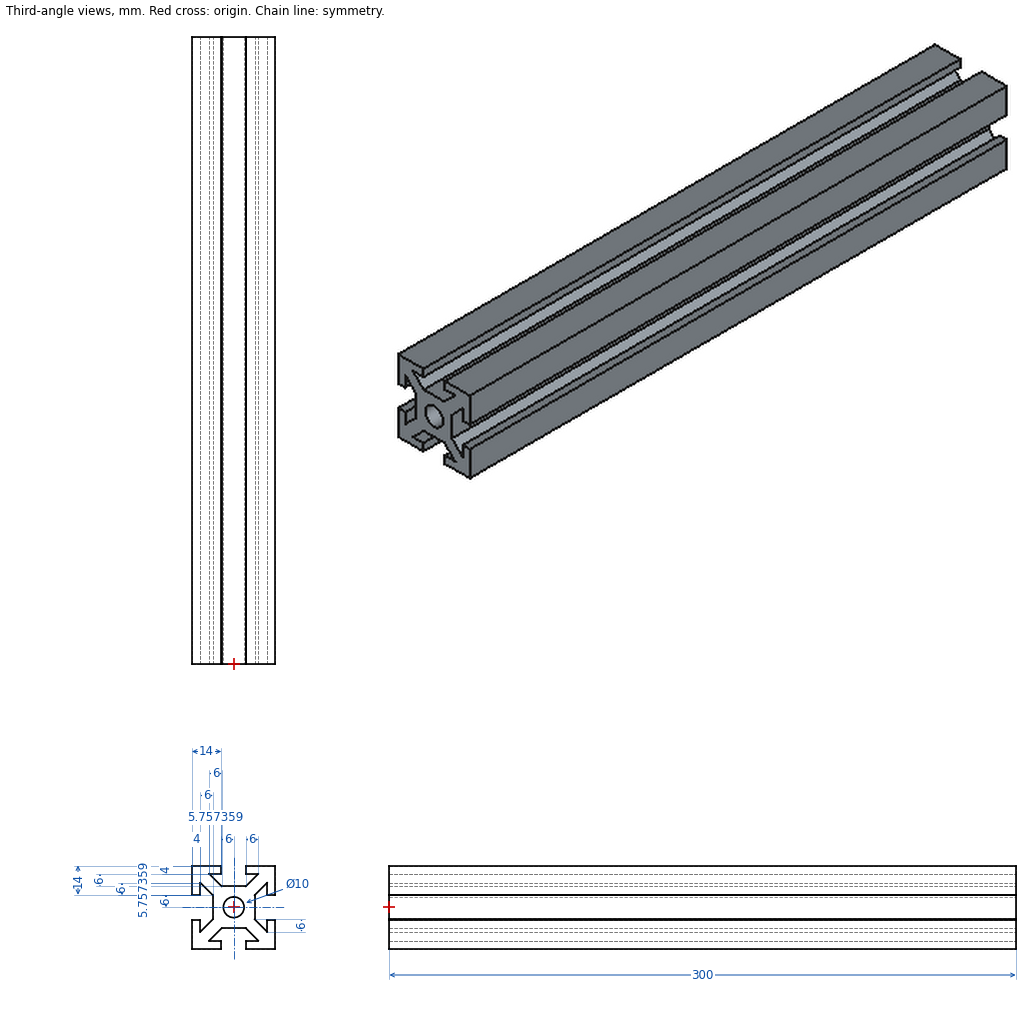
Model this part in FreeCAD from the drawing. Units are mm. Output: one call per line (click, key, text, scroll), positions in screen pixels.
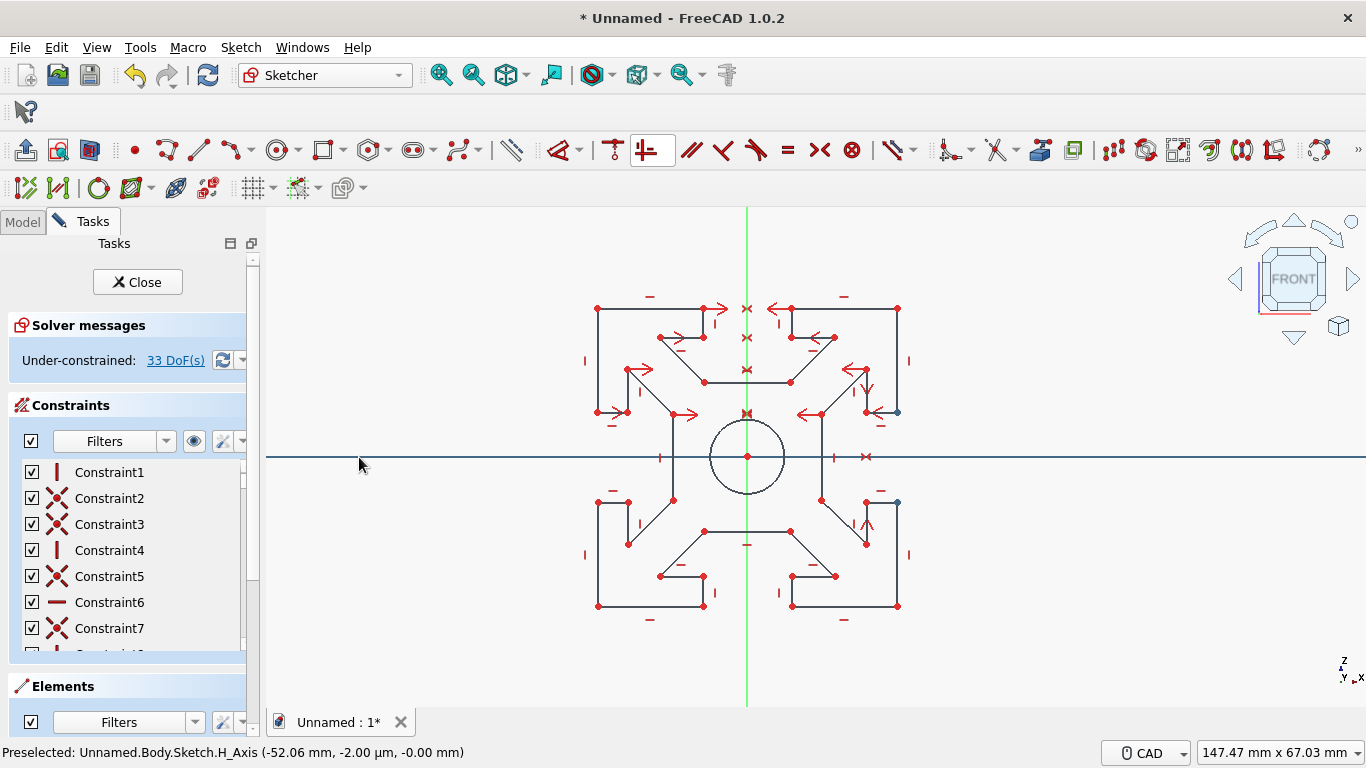
key(s)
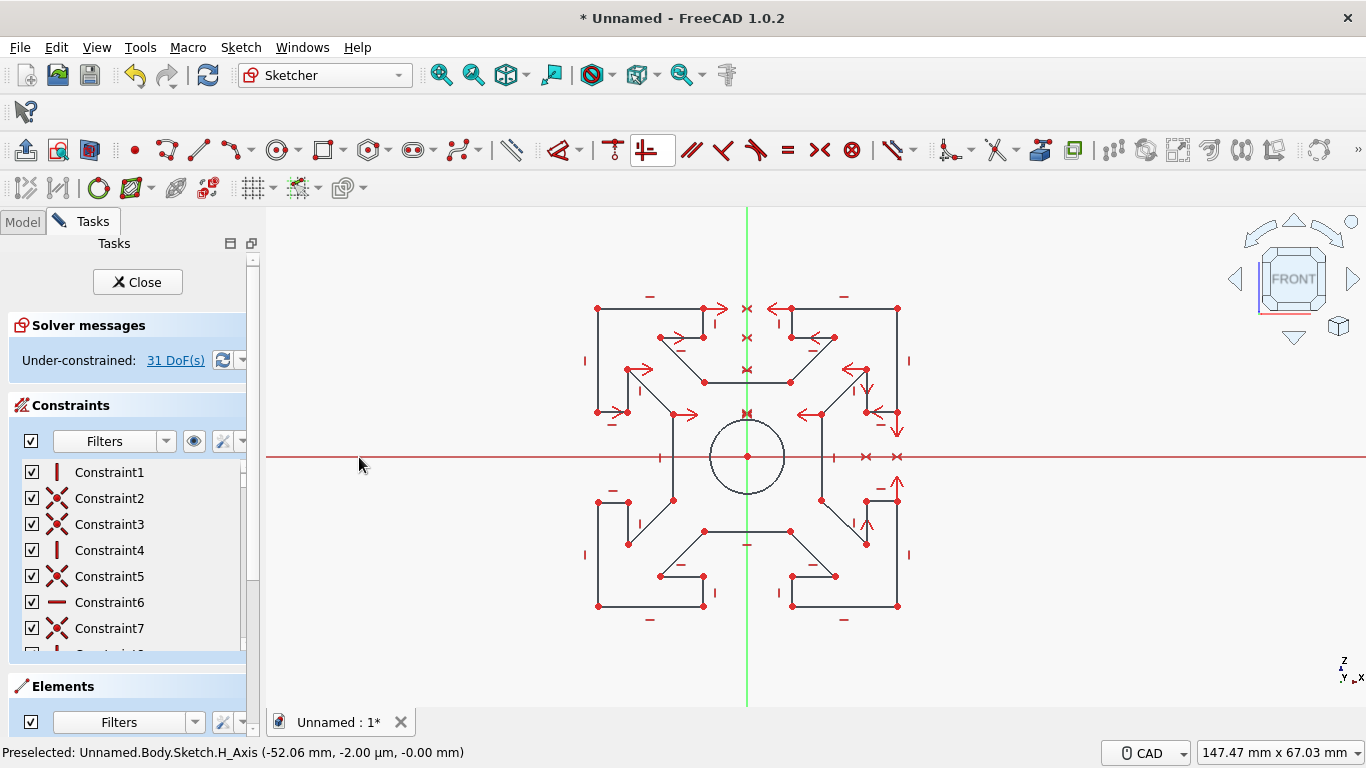
click(792, 309)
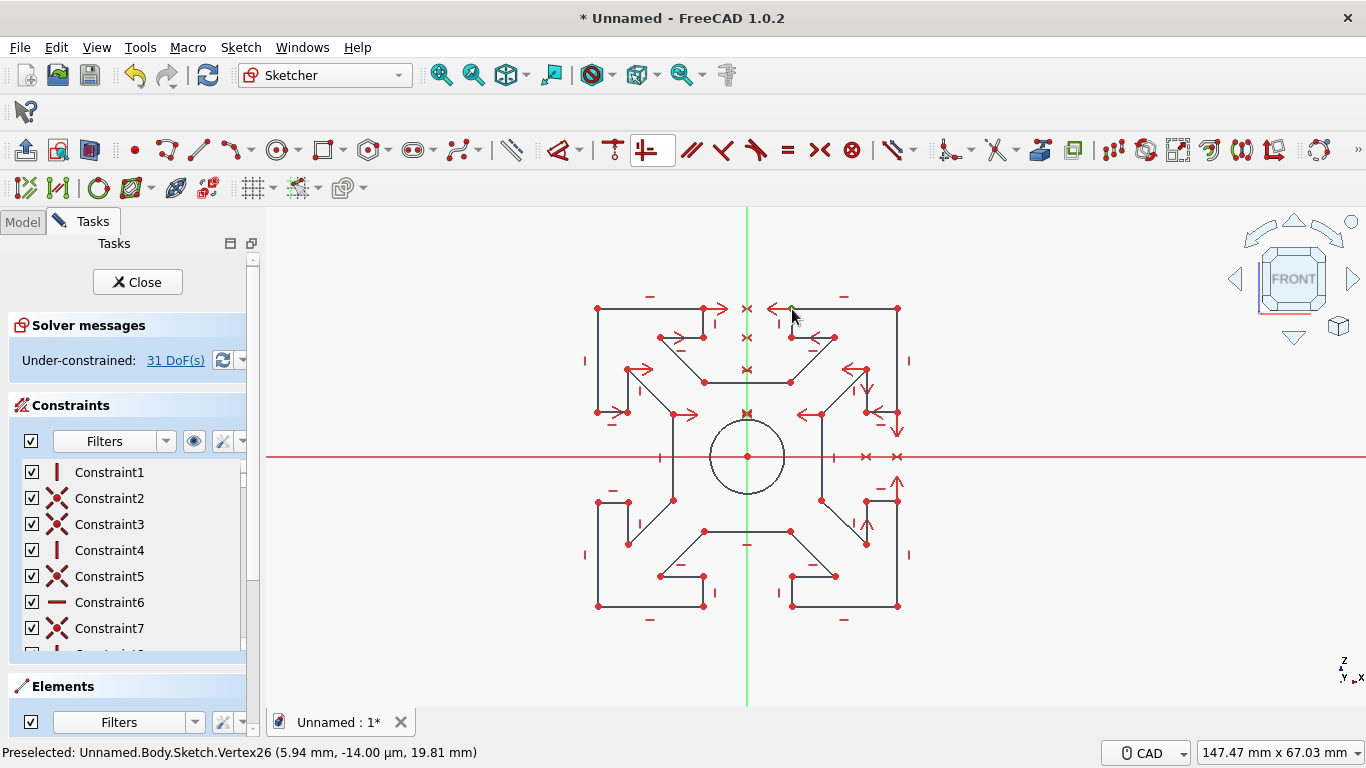
click(792, 607)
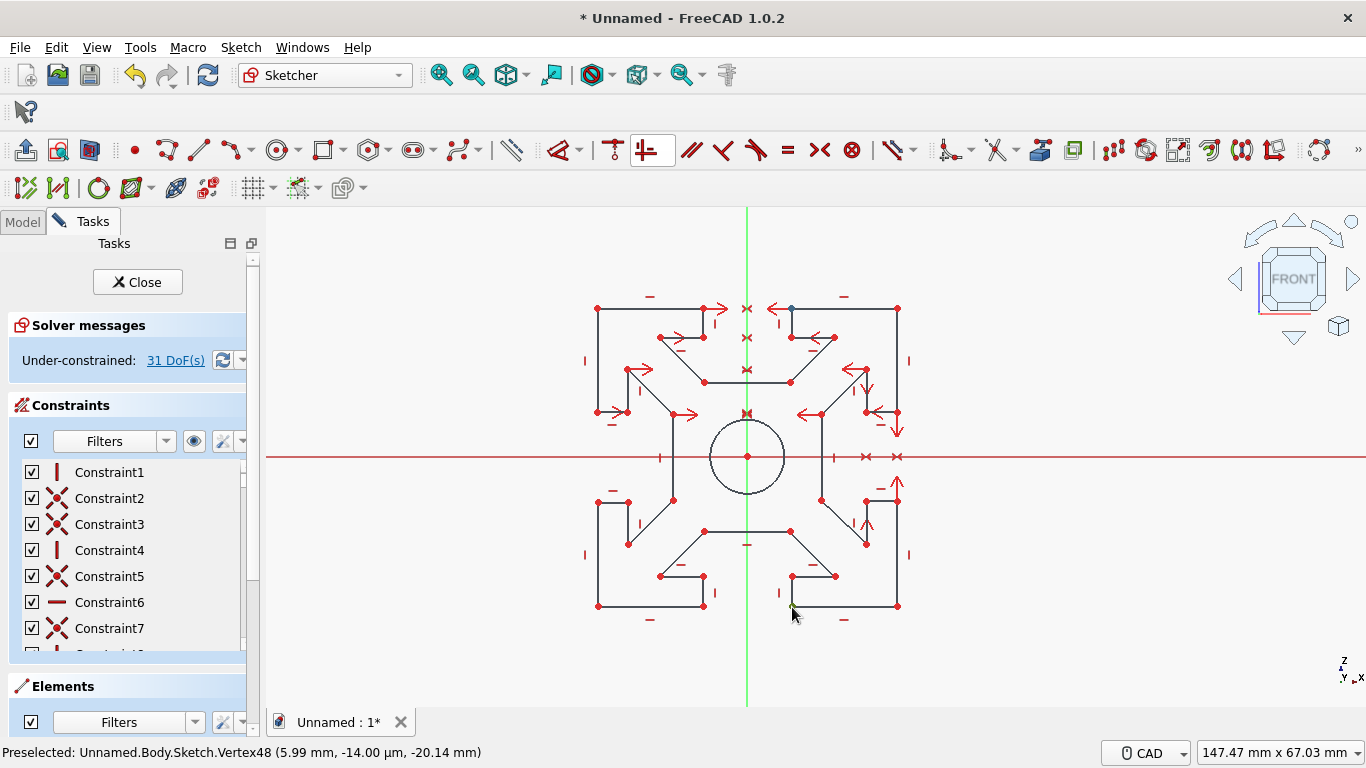
click(359, 457)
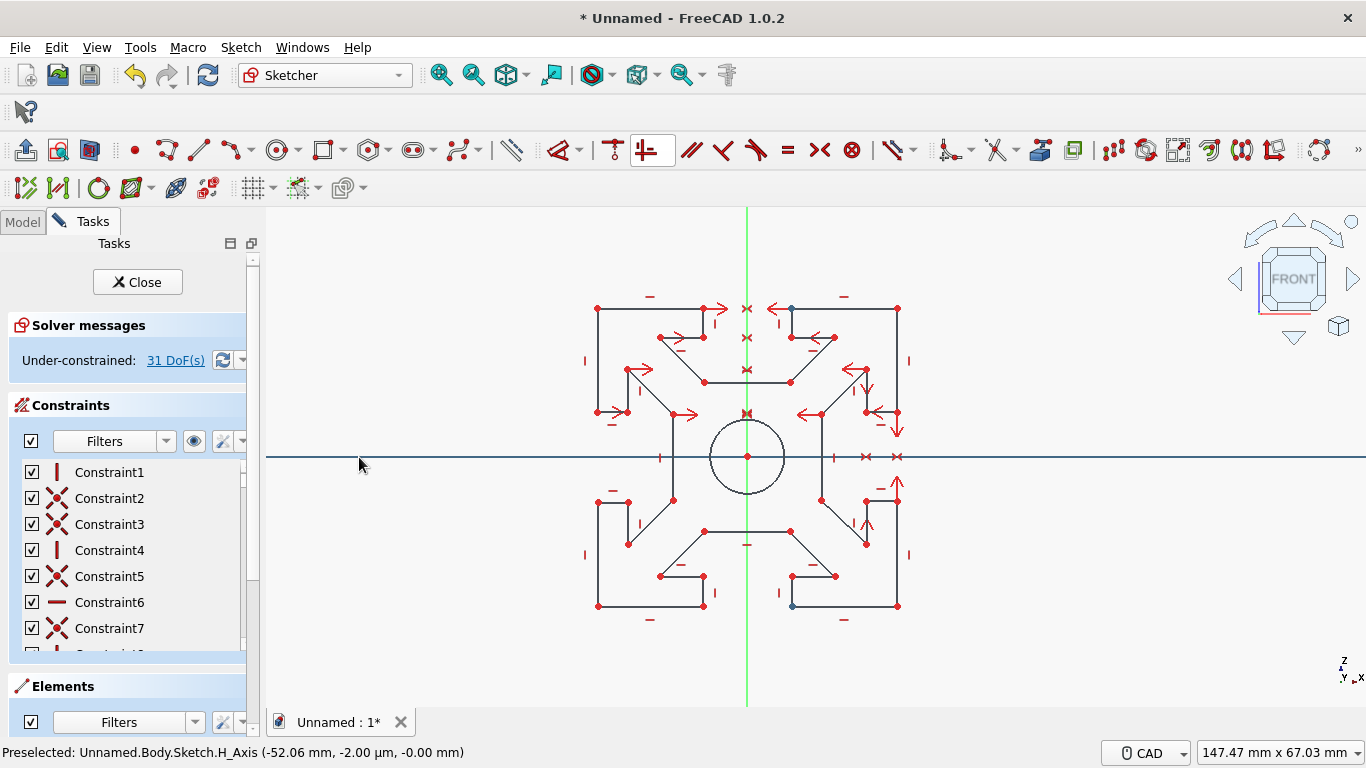
key(s)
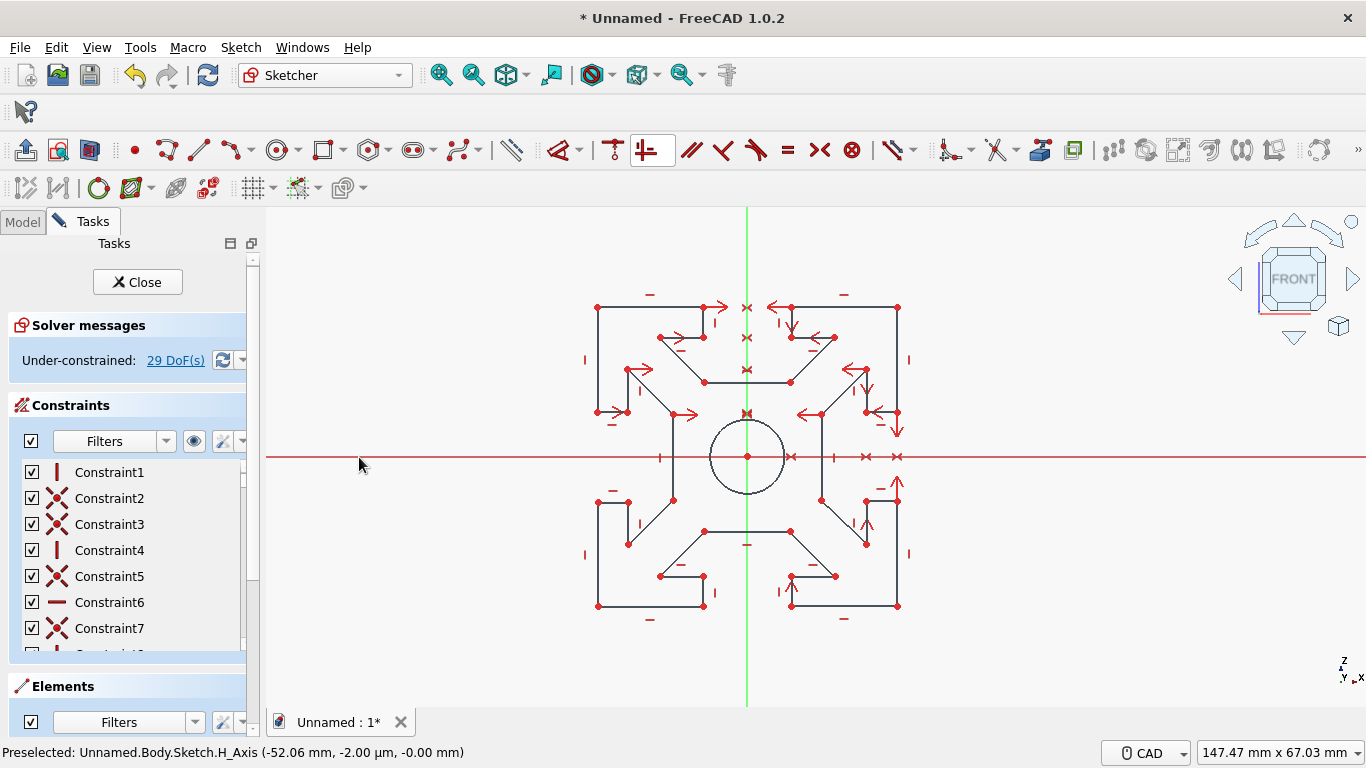
click(835, 338)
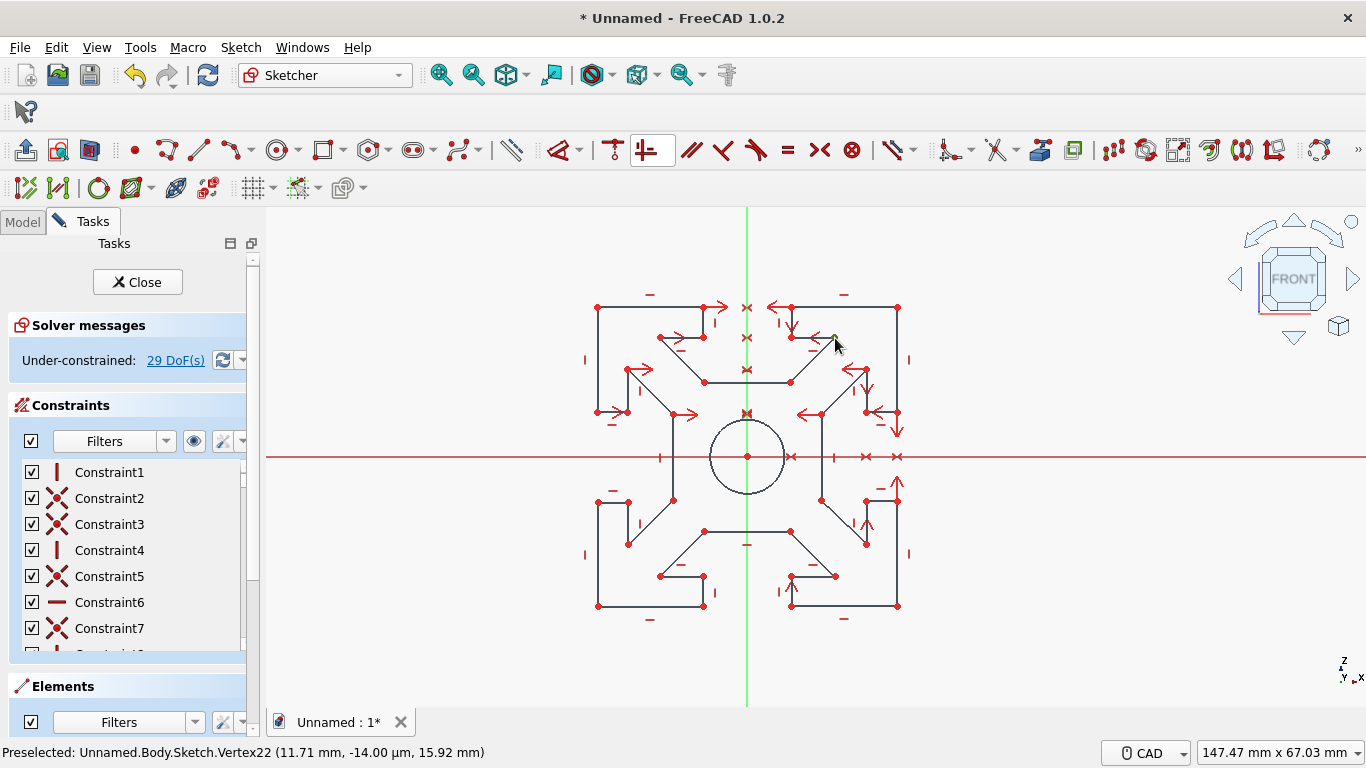
click(835, 577)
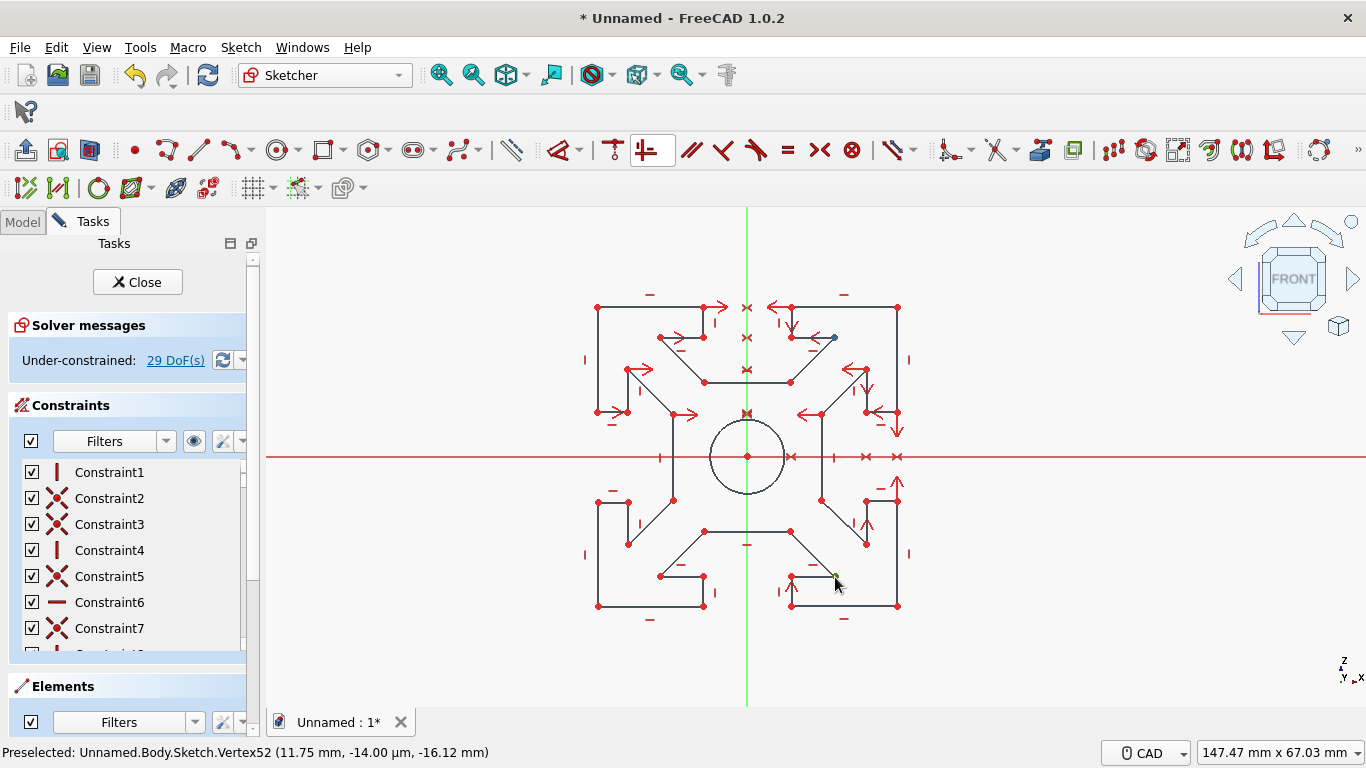
click(359, 457)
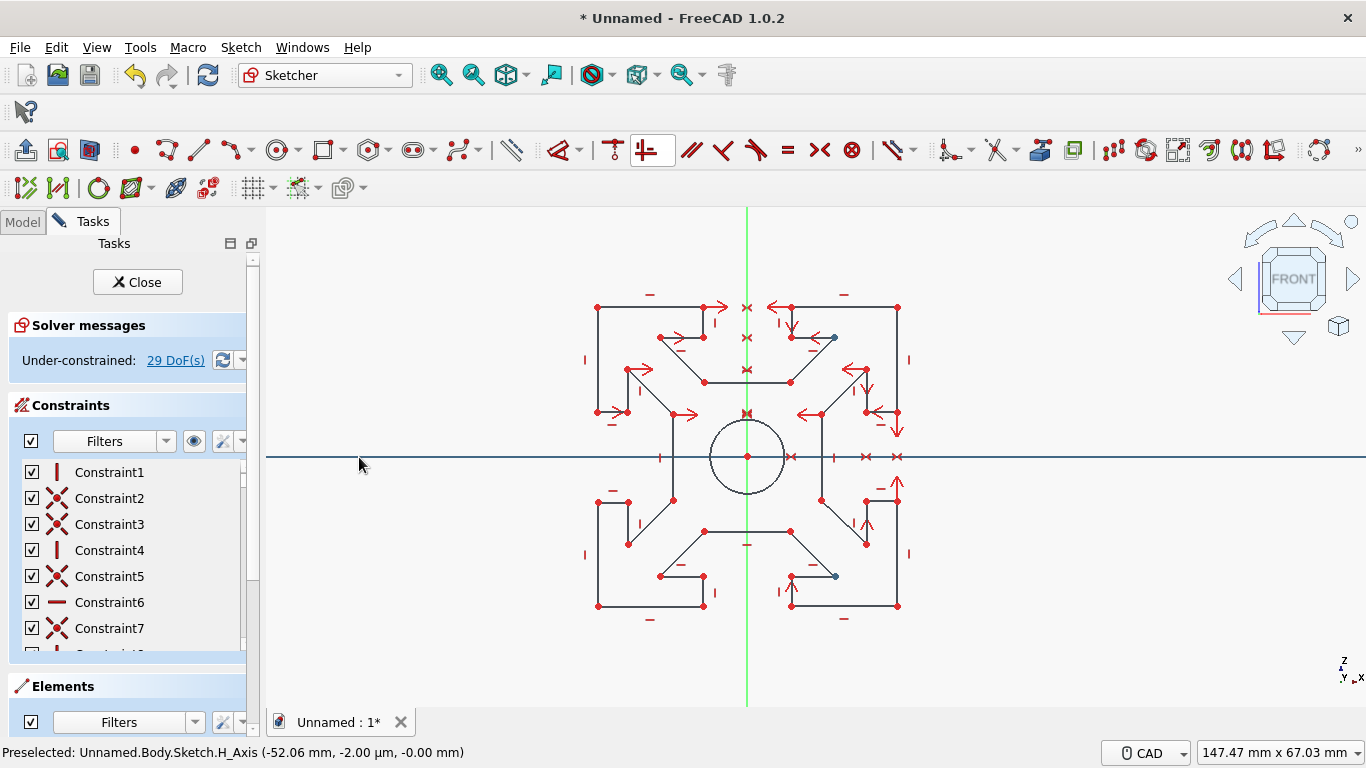
click(820, 150)